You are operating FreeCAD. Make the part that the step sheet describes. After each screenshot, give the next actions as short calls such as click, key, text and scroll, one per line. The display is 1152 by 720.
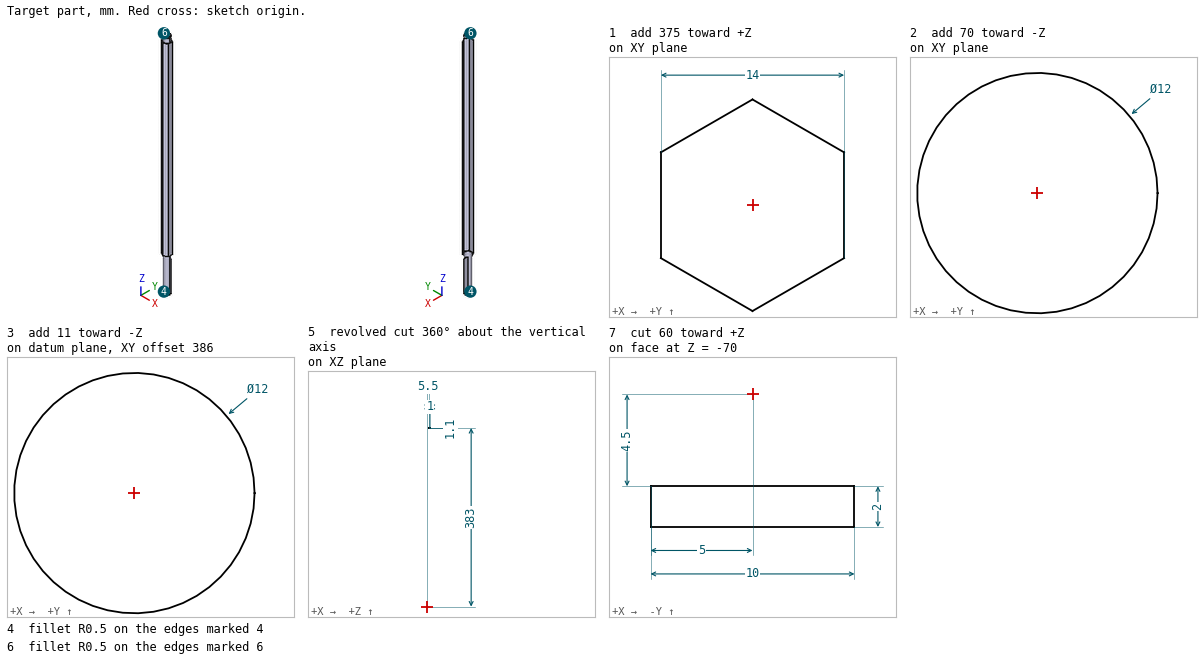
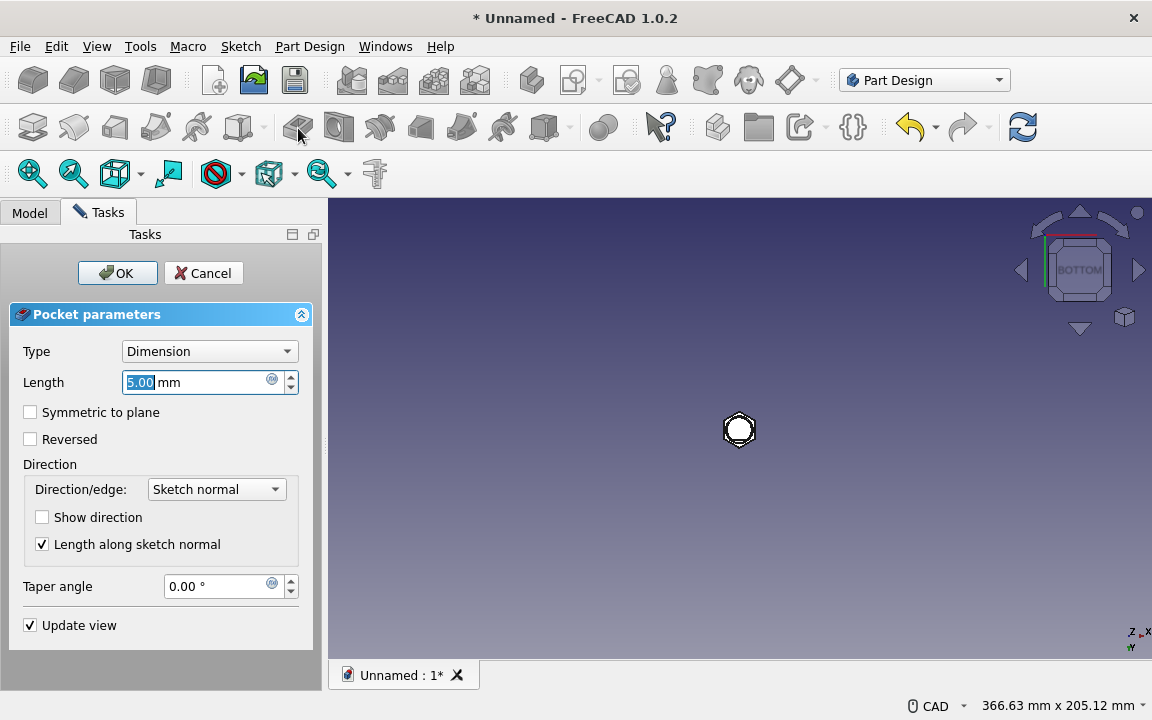
text(60)
key(Tab)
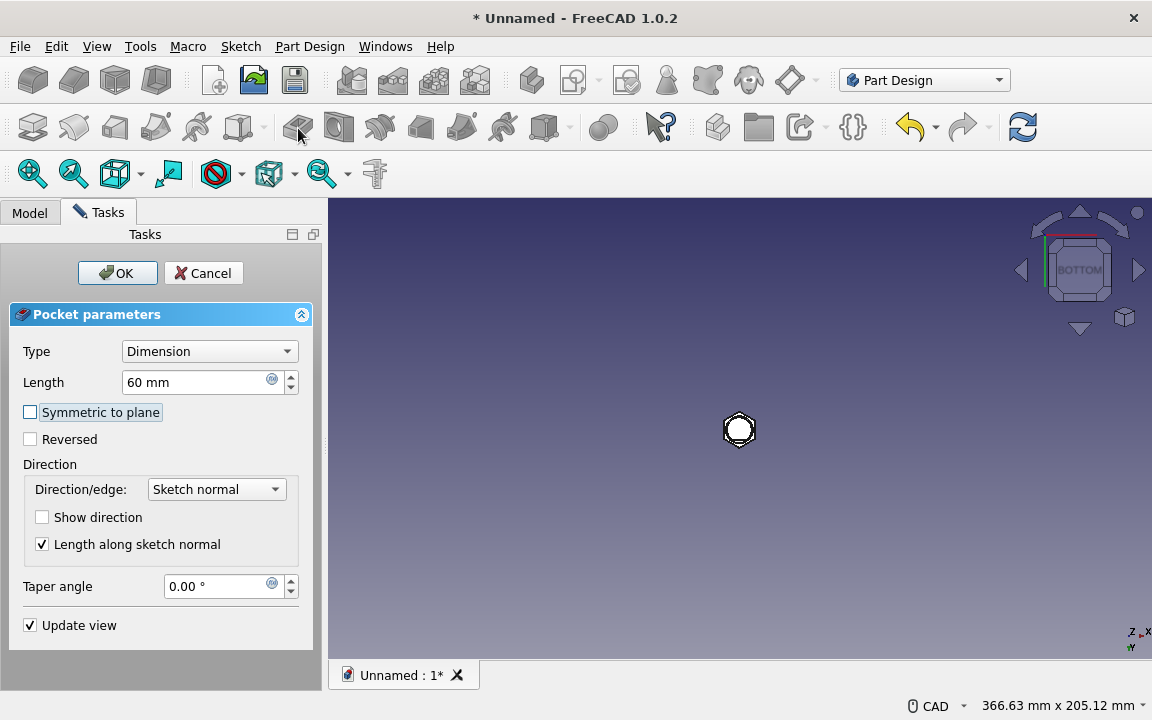
click(118, 273)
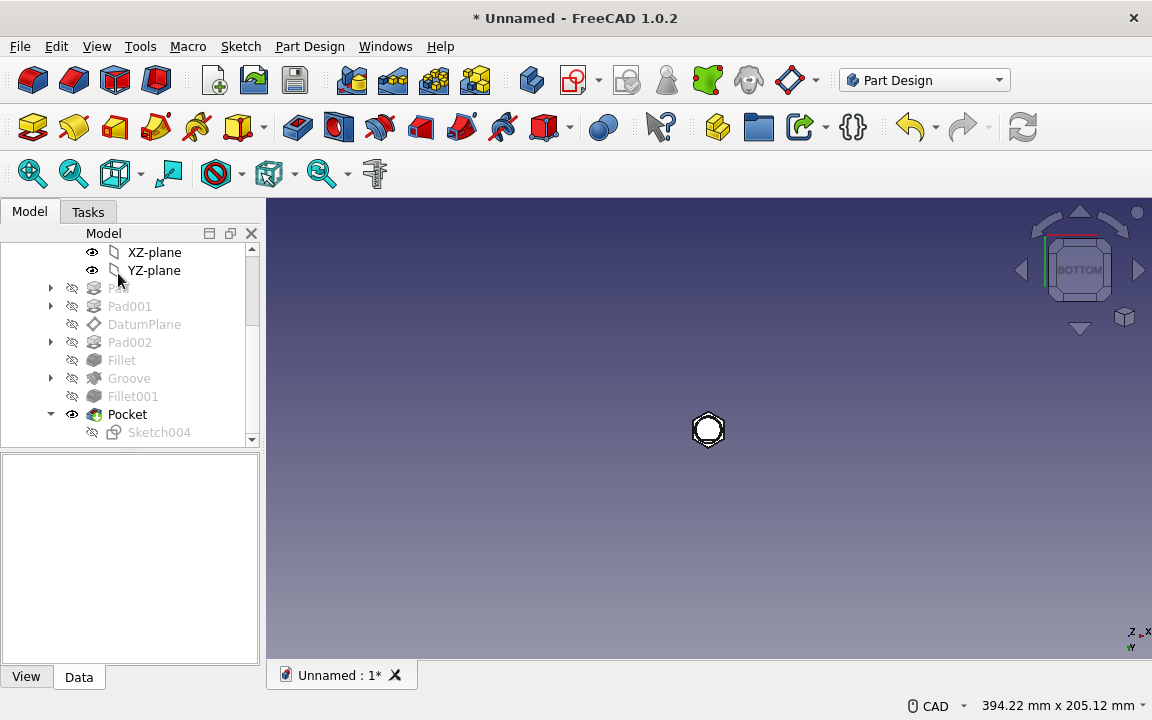
key(0)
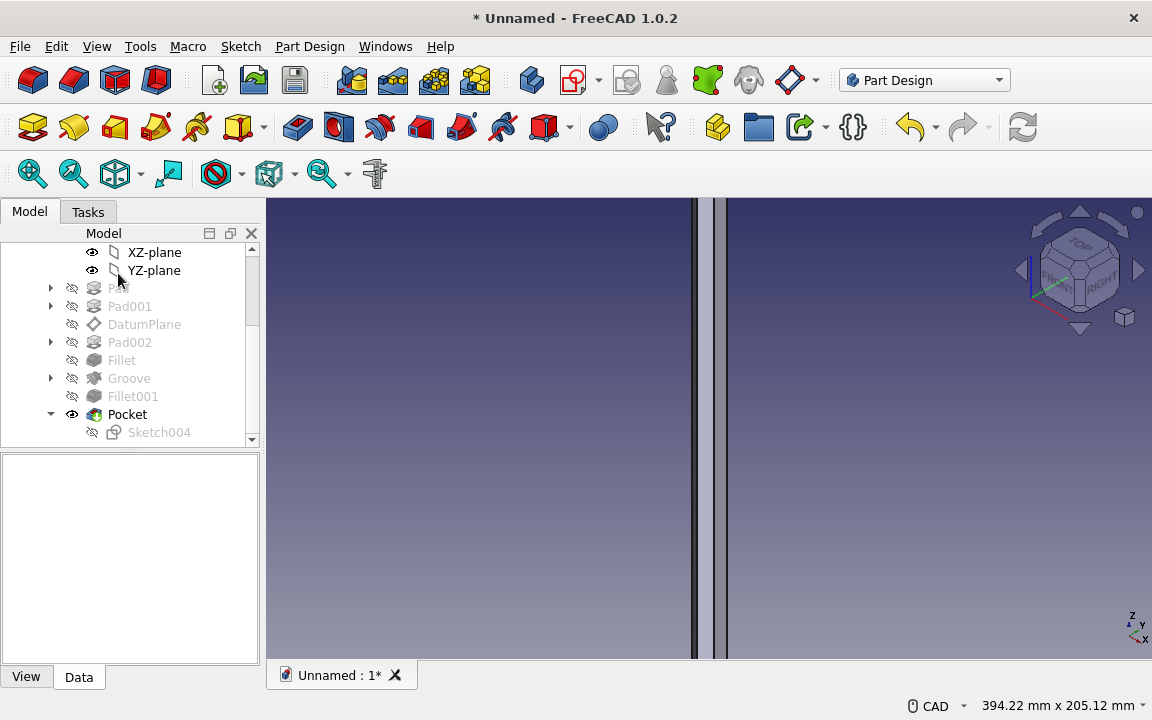
click(33, 174)